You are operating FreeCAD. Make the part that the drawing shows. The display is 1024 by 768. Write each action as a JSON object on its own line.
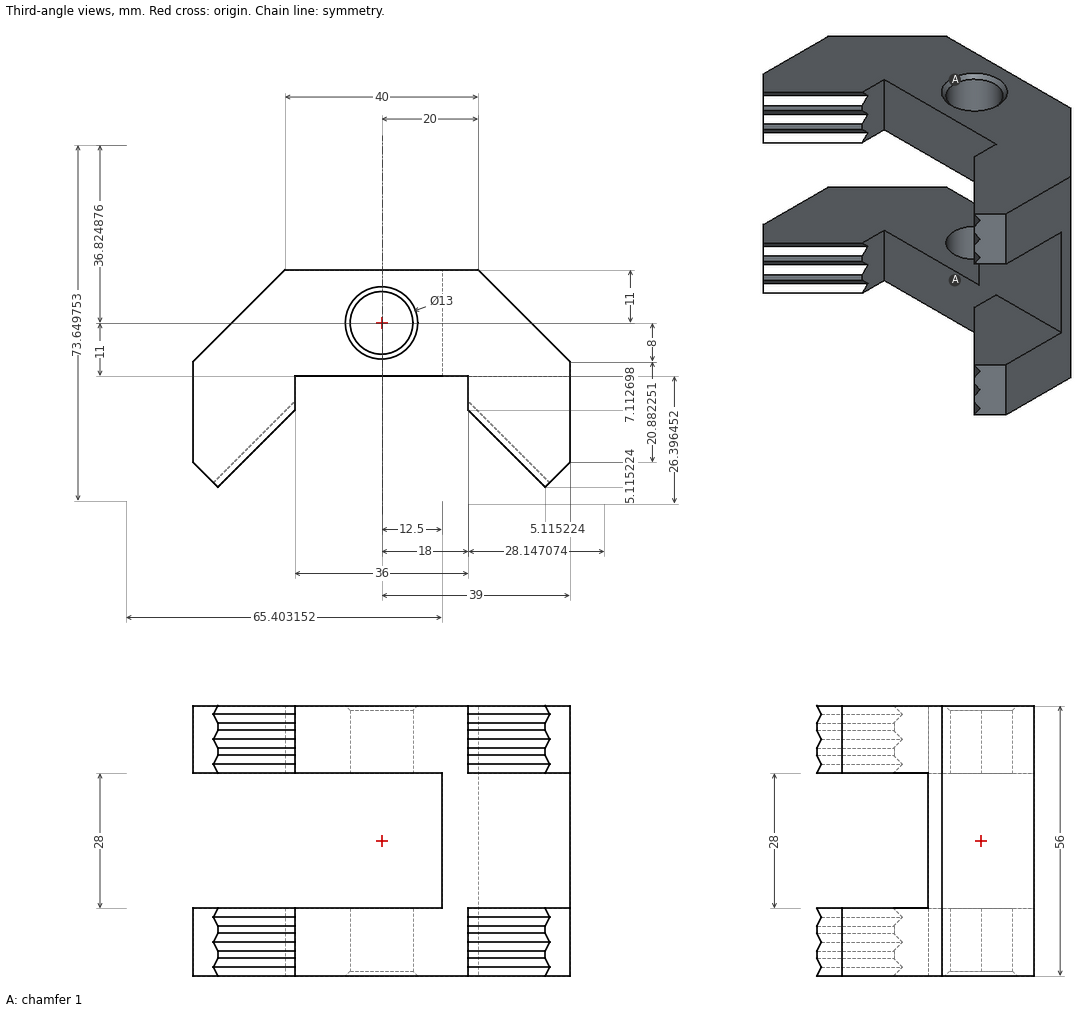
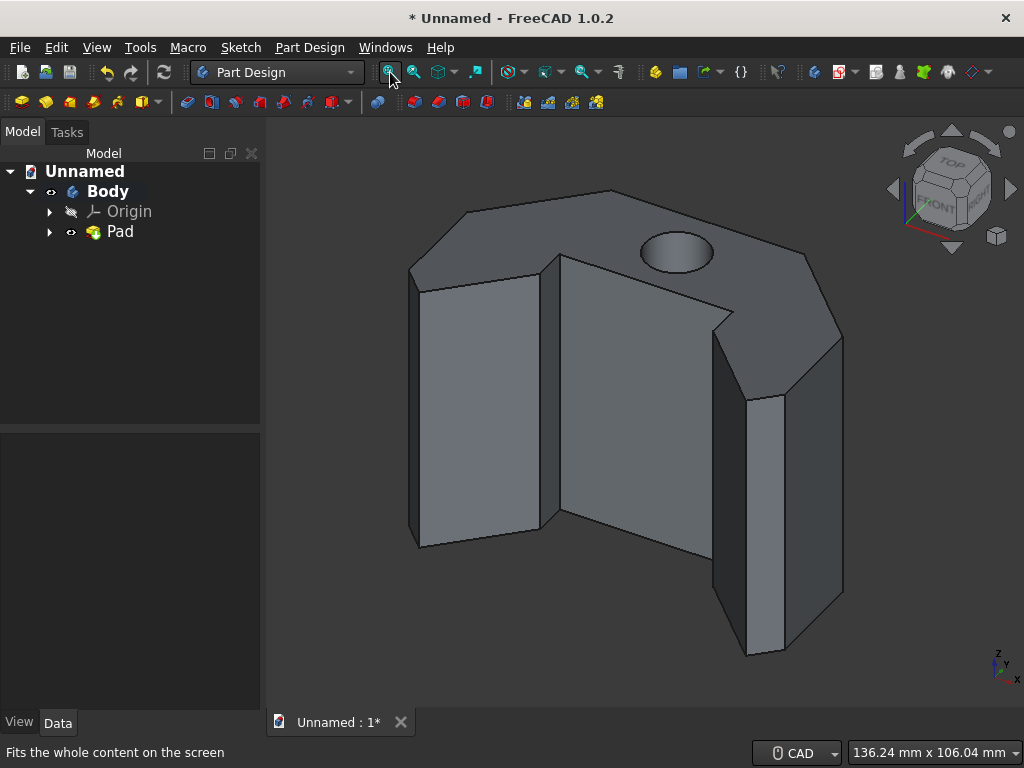
{"action": "left_click", "coordinate": [50, 212]}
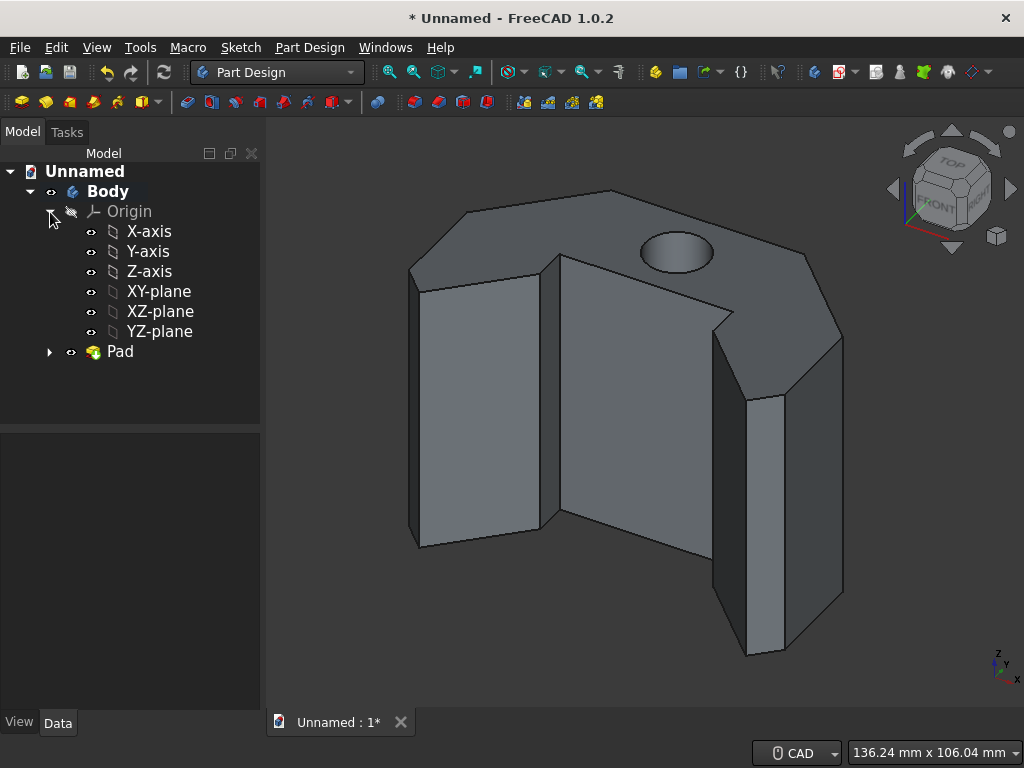
{"action": "left_click", "coordinate": [136, 292]}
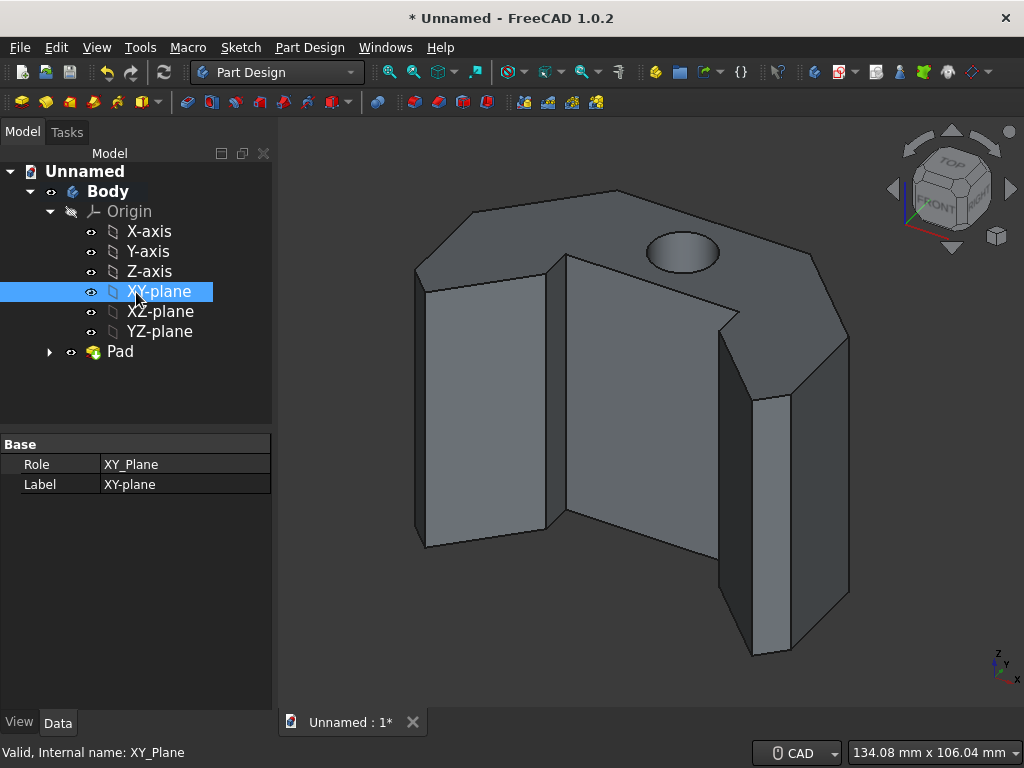
{"action": "left_click", "coordinate": [972, 72]}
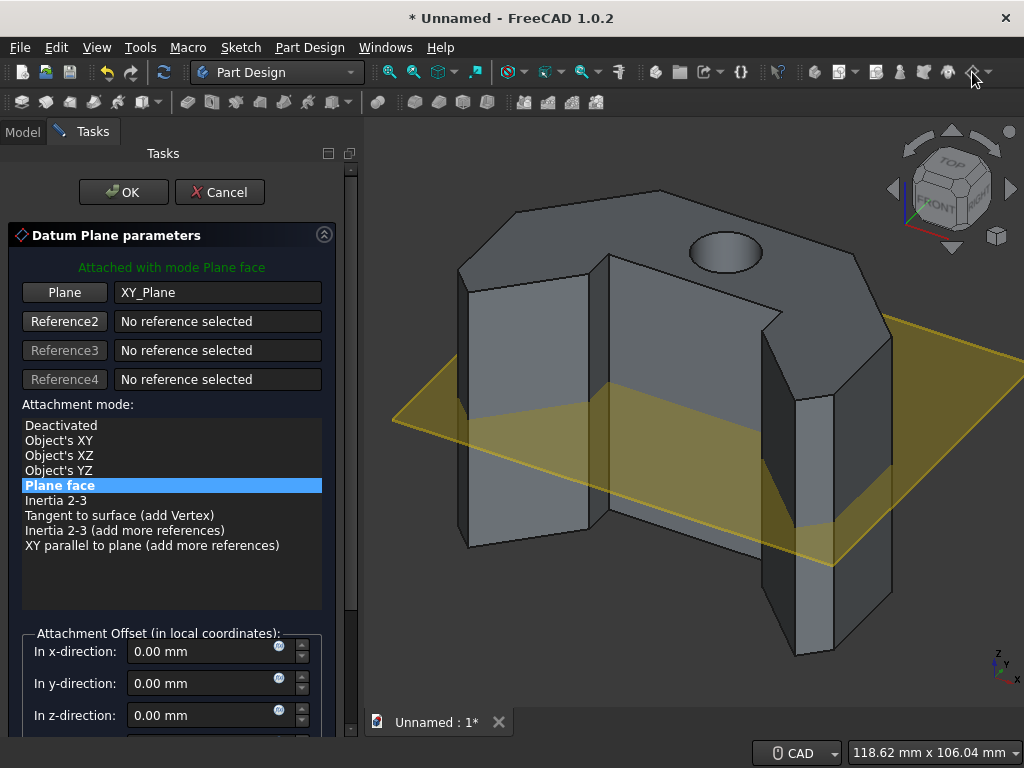
{"action": "triple_click", "coordinate": [210, 715]}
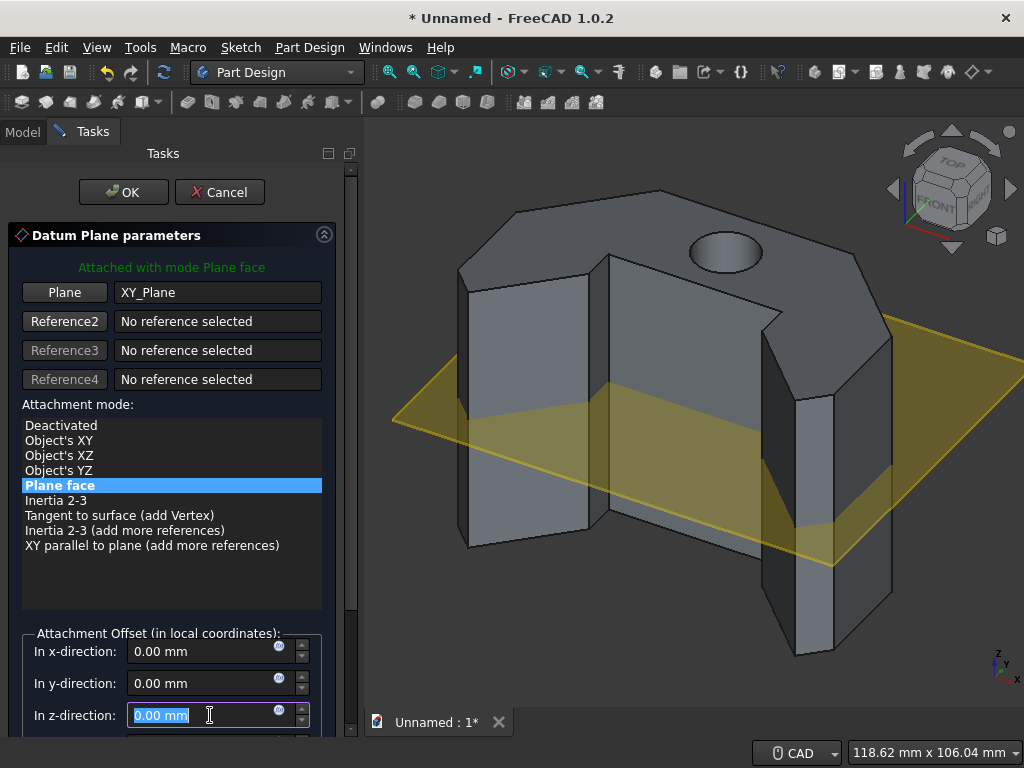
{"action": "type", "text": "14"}
{"action": "key", "text": "Tab"}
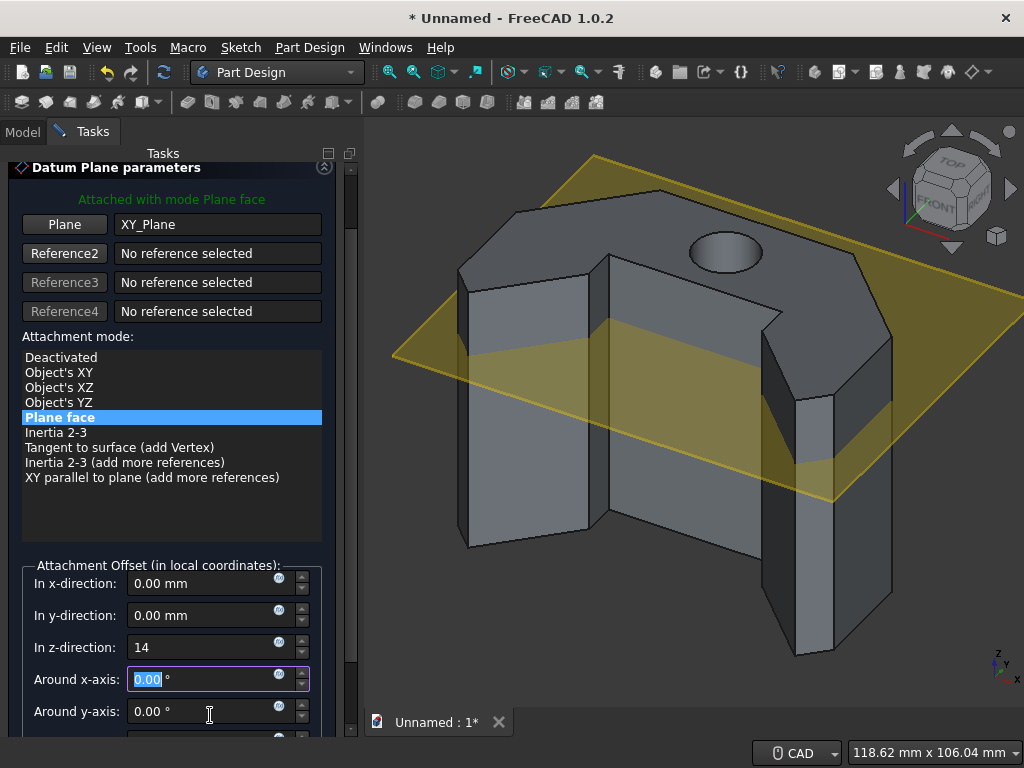
{"action": "scroll", "coordinate": [351, 450], "scroll_direction": "up", "scroll_amount": 2}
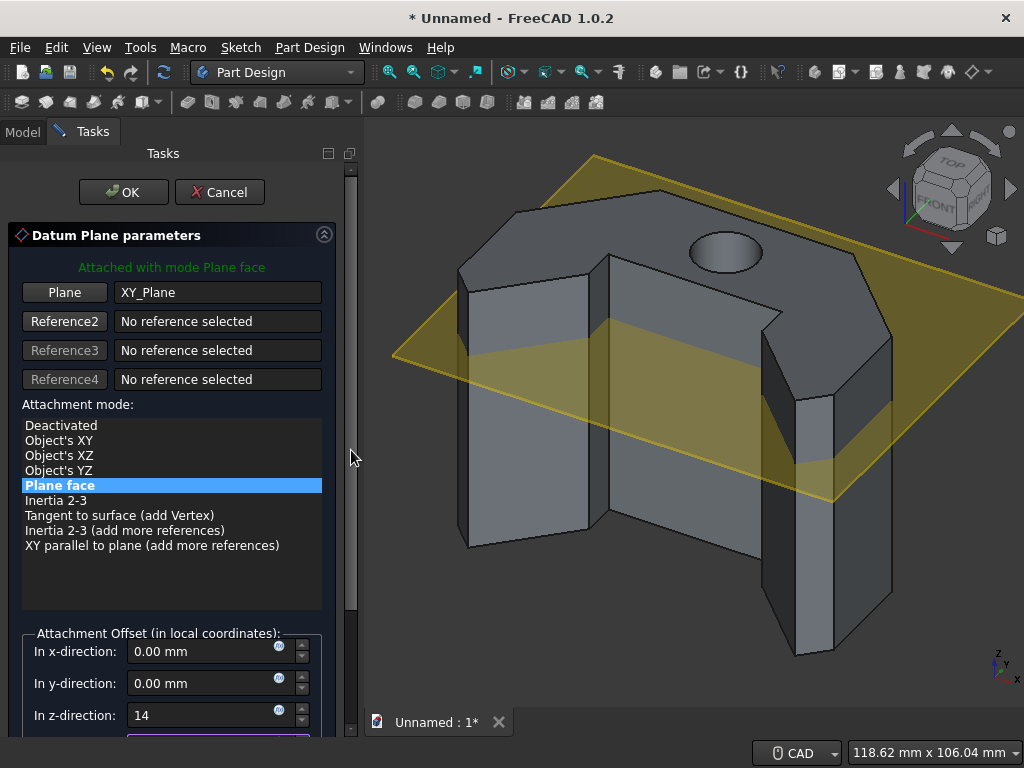
{"action": "left_click", "coordinate": [124, 192]}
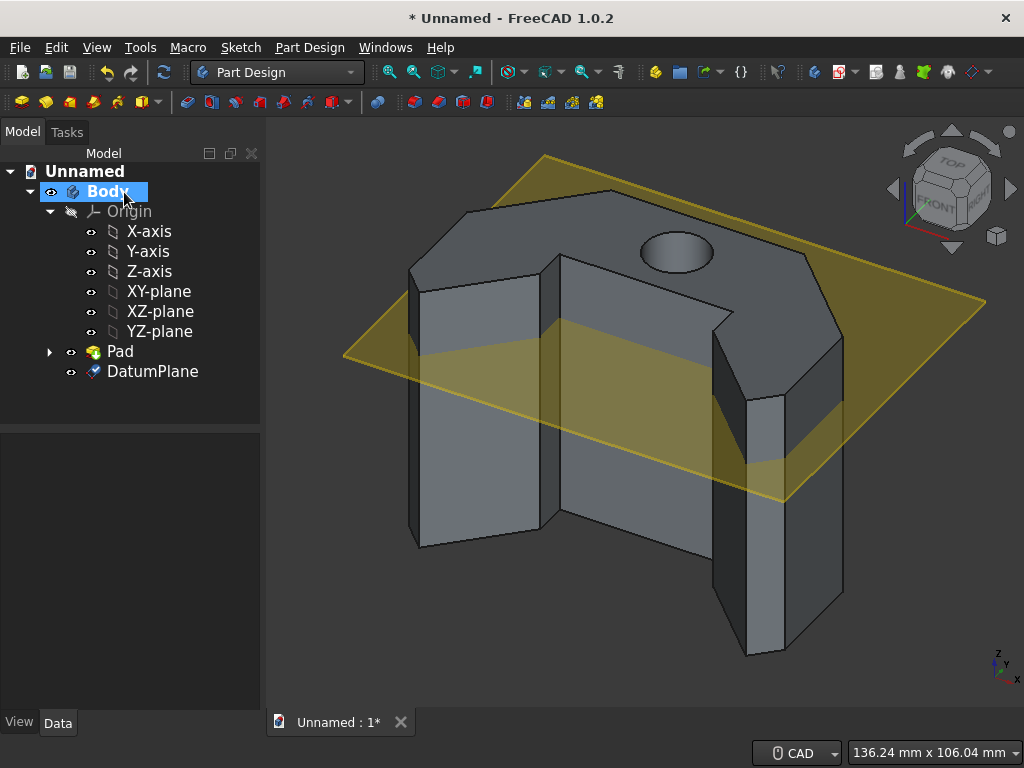
{"action": "left_click", "coordinate": [116, 372]}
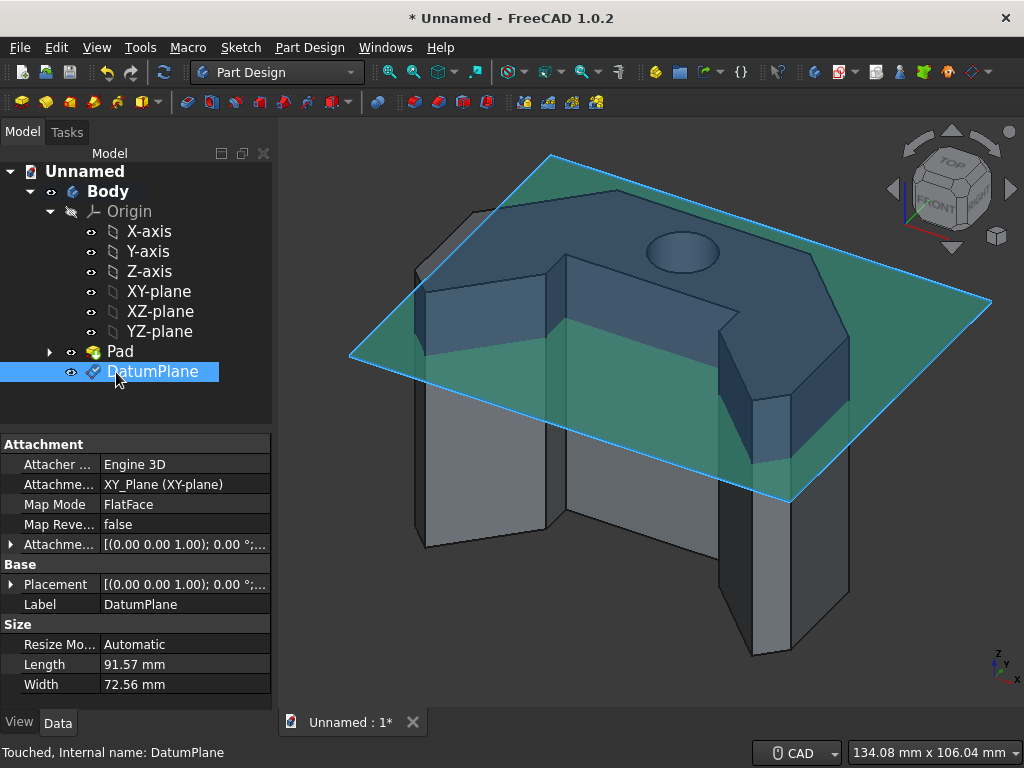
{"action": "left_click", "coordinate": [840, 72]}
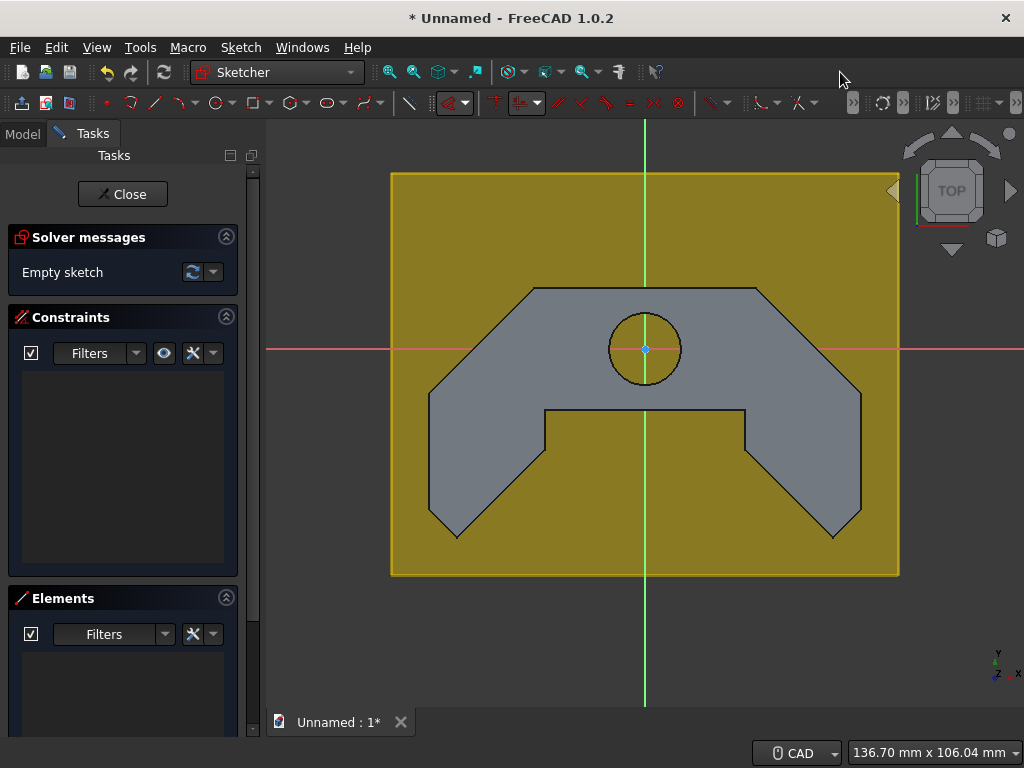
{"action": "left_click", "coordinate": [70, 104]}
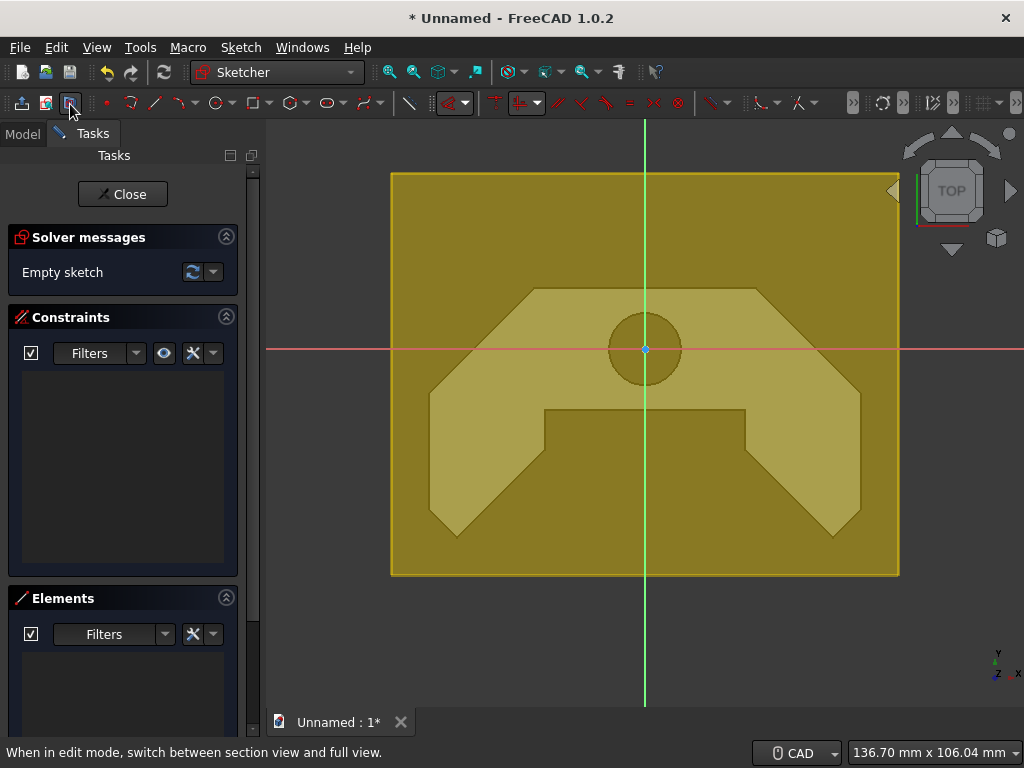
{"action": "scroll", "coordinate": [773, 679], "scroll_direction": "down", "scroll_amount": 1}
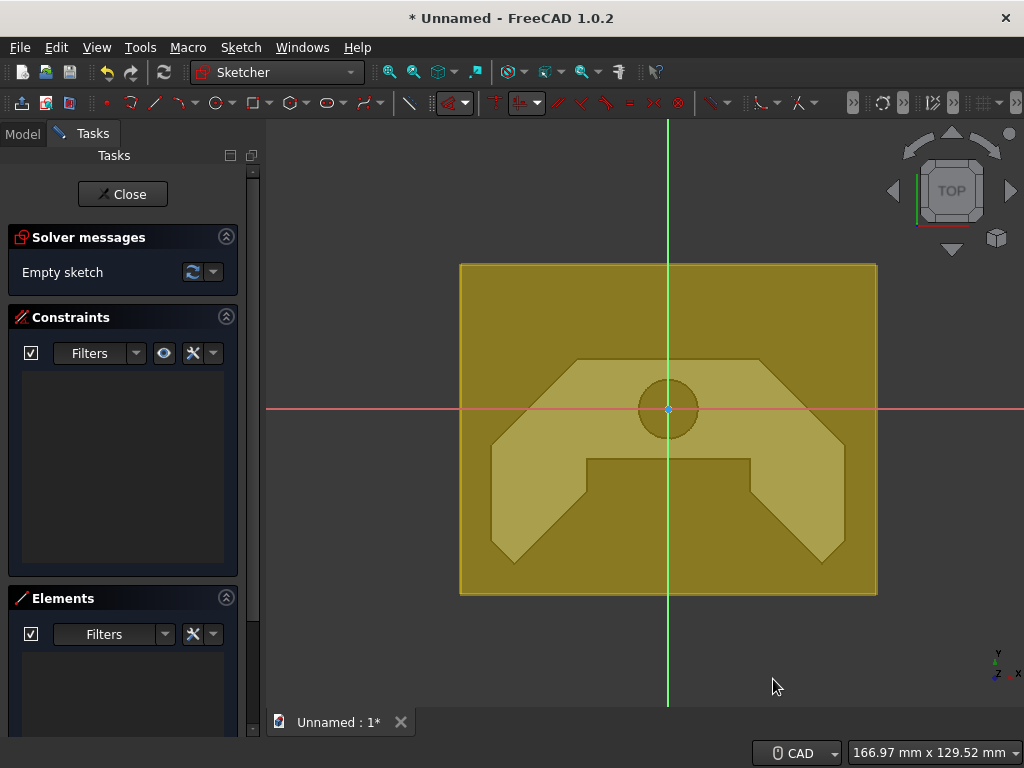
{"action": "left_click", "coordinate": [254, 104]}